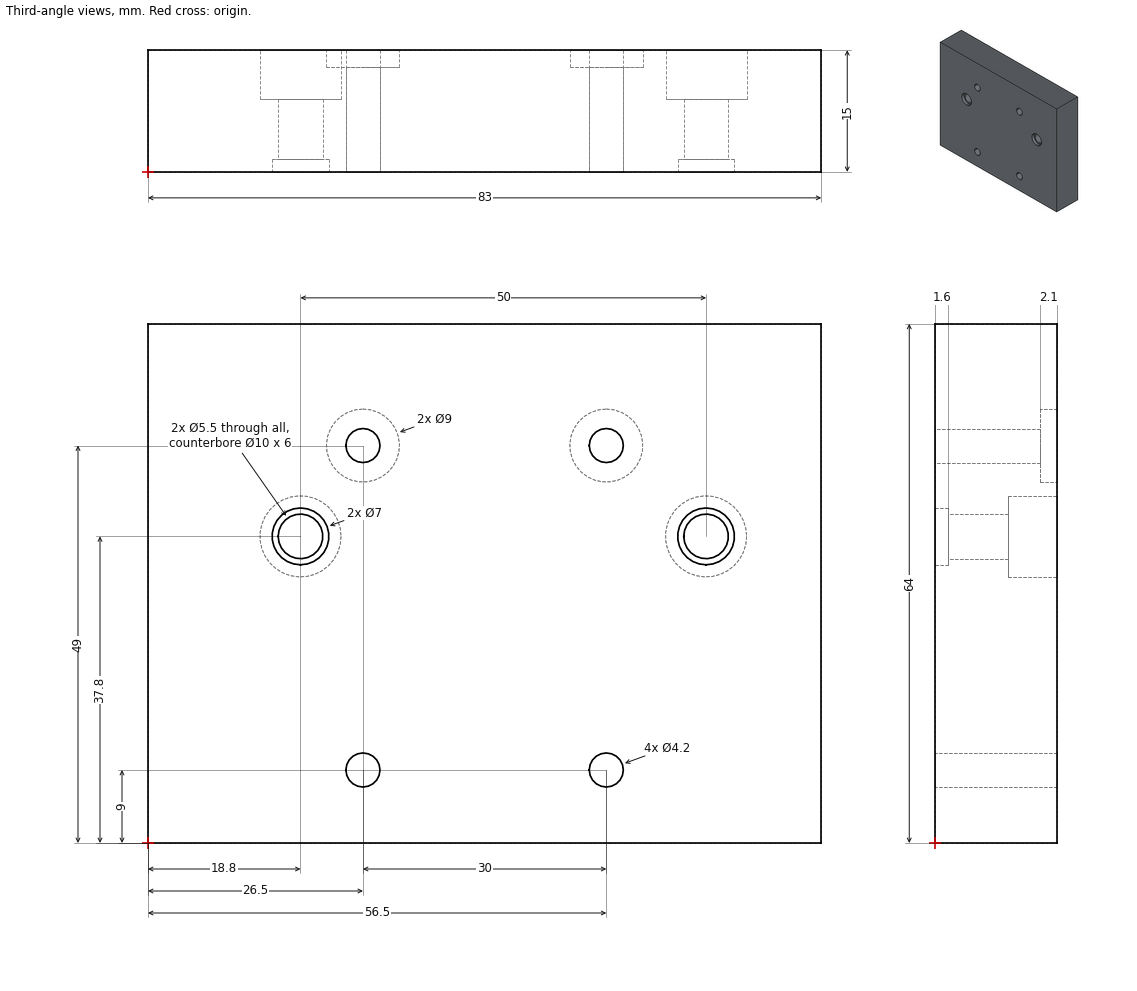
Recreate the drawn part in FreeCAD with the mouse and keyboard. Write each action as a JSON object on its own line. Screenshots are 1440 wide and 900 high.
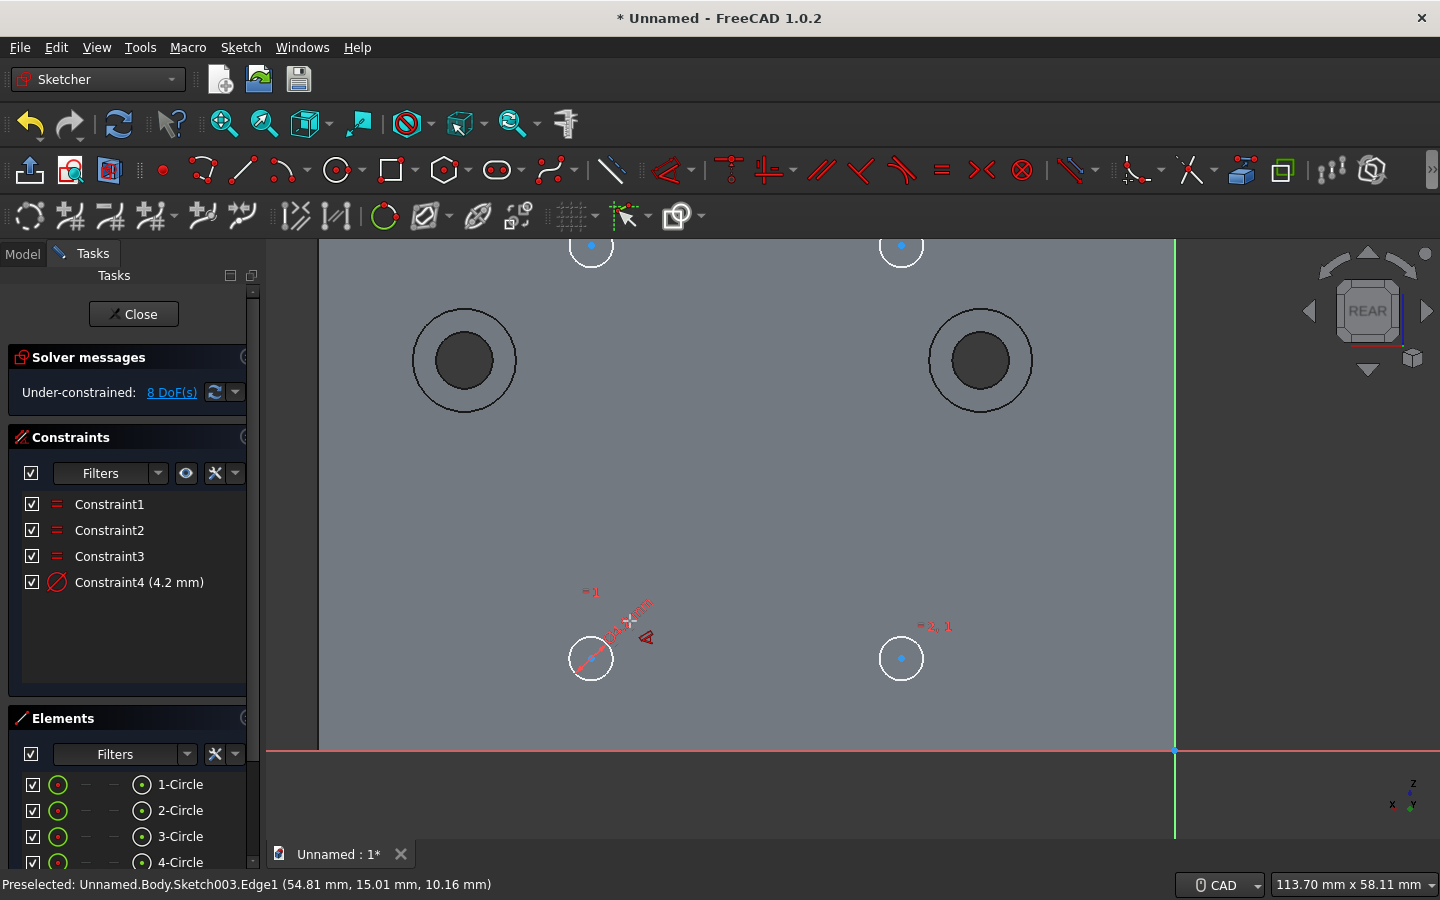
{"action": "left_click", "coordinate": [591, 659]}
{"action": "left_click", "coordinate": [1209, 705]}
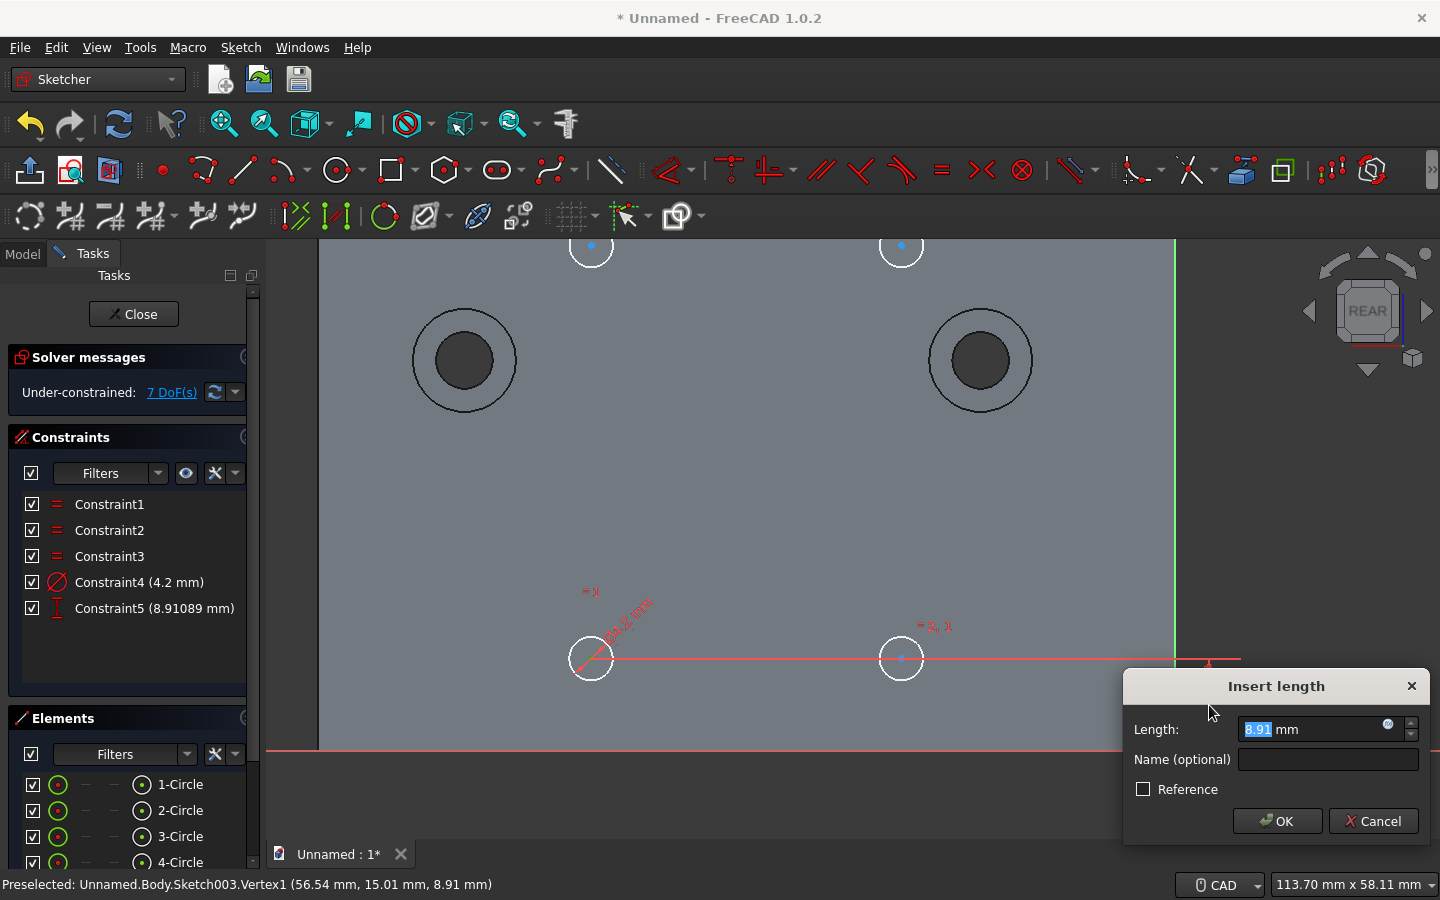
{"action": "type", "text": "9"}
{"action": "key", "text": "Return"}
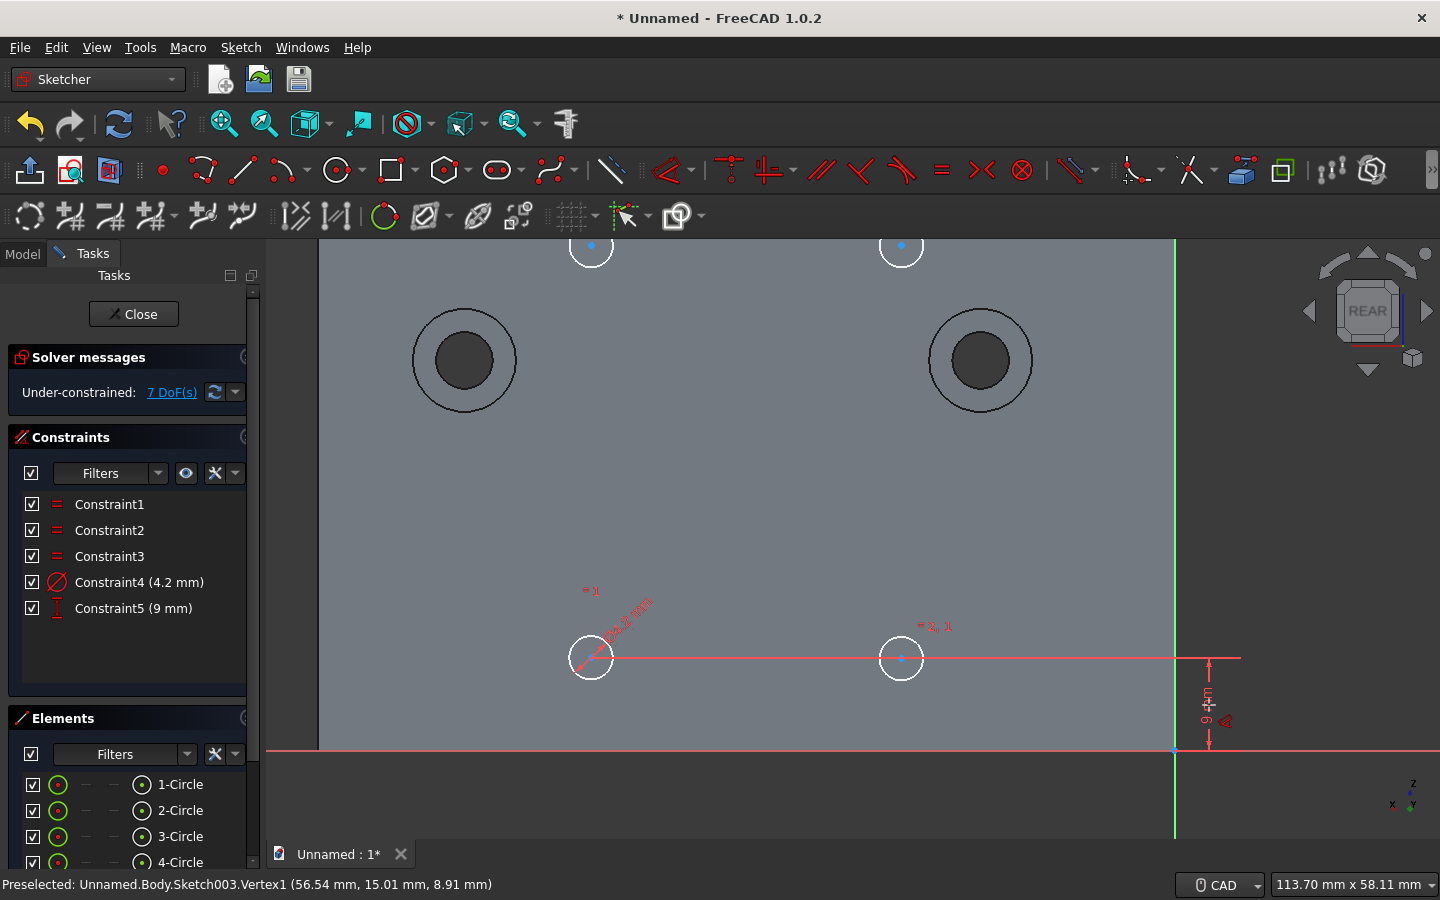
{"action": "left_click", "coordinate": [901, 659]}
{"action": "left_click", "coordinate": [1209, 684]}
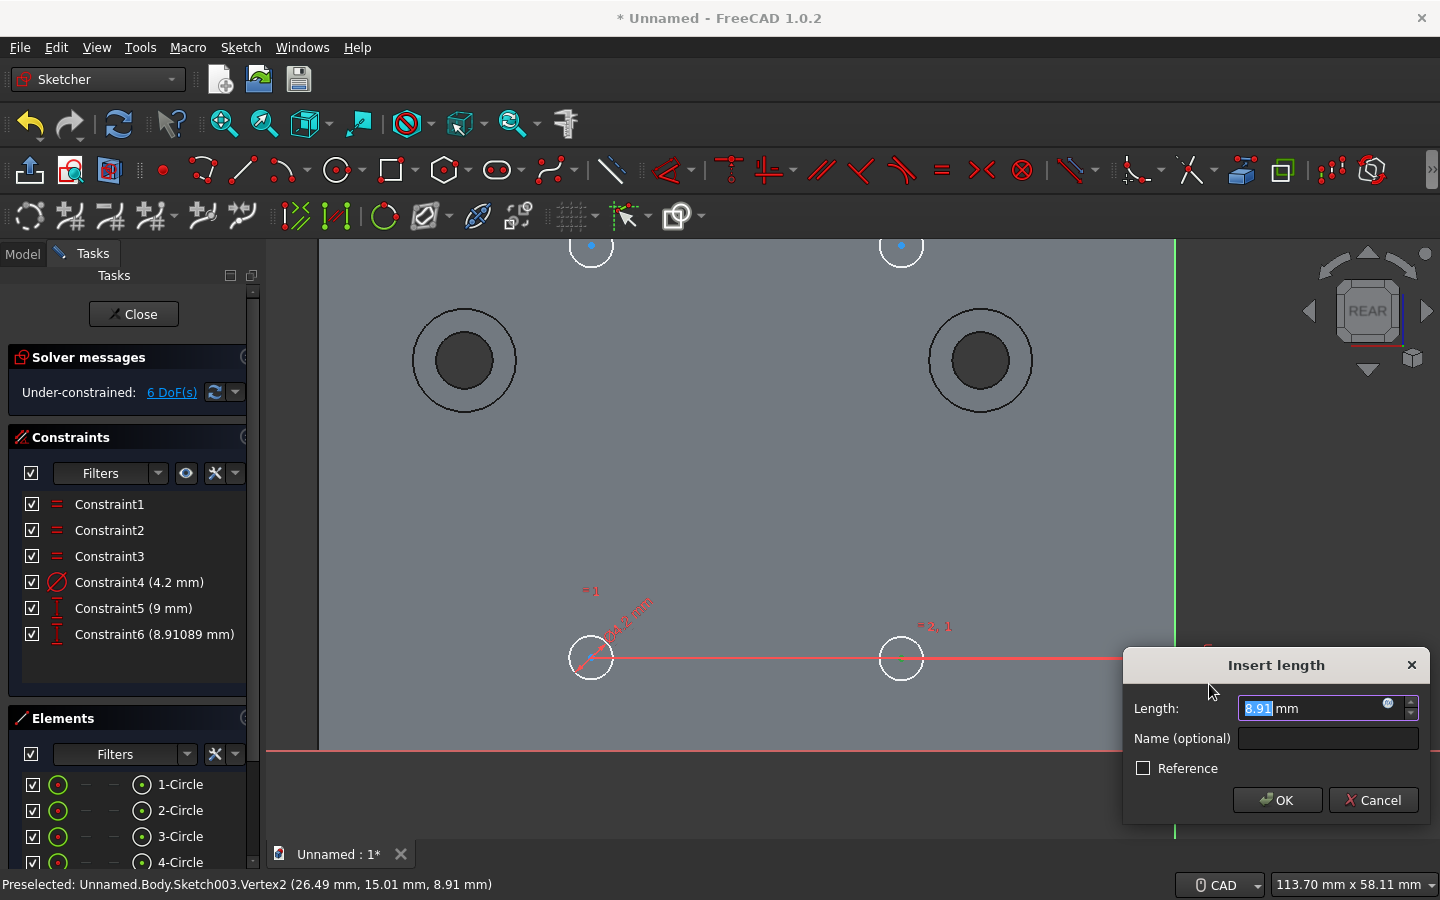
{"action": "type", "text": "9"}
{"action": "key", "text": "Return"}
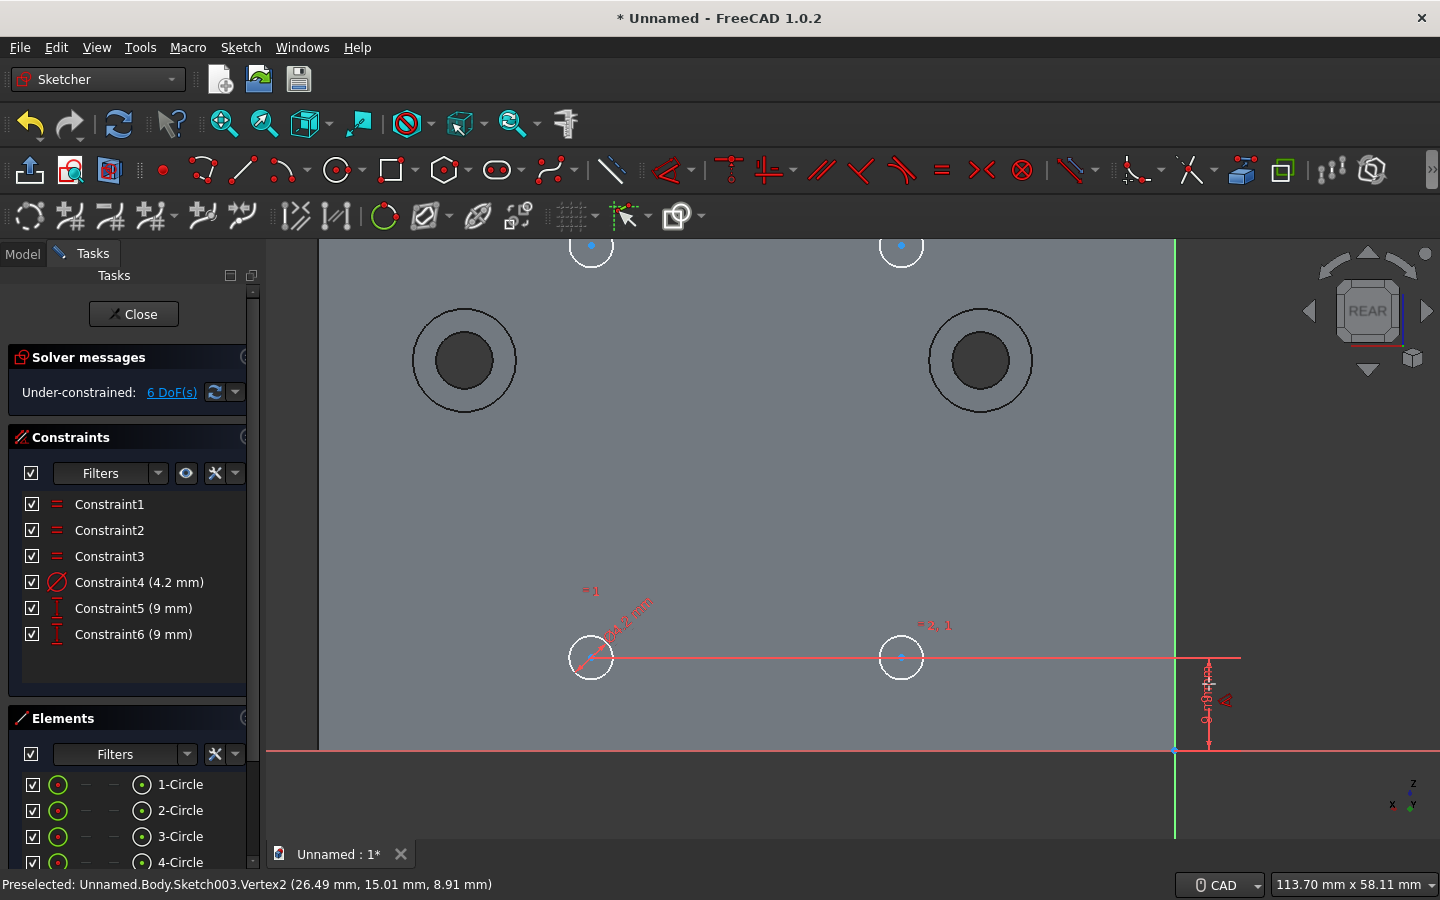
{"action": "scroll", "coordinate": [606, 645], "scroll_direction": "down", "scroll_amount": 2}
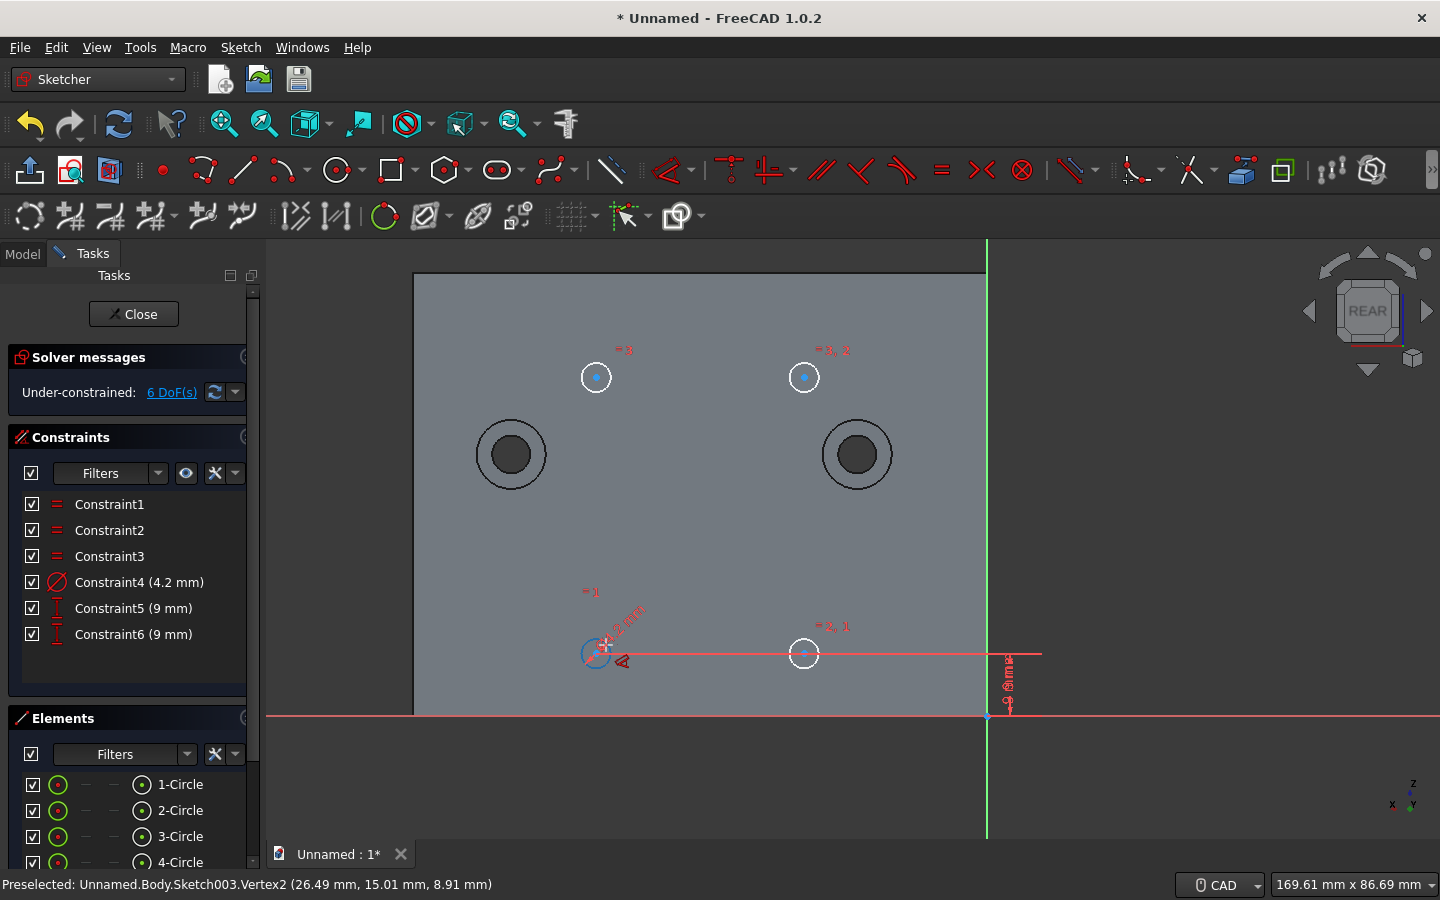
{"action": "left_click", "coordinate": [804, 378]}
{"action": "left_click", "coordinate": [1021, 547]}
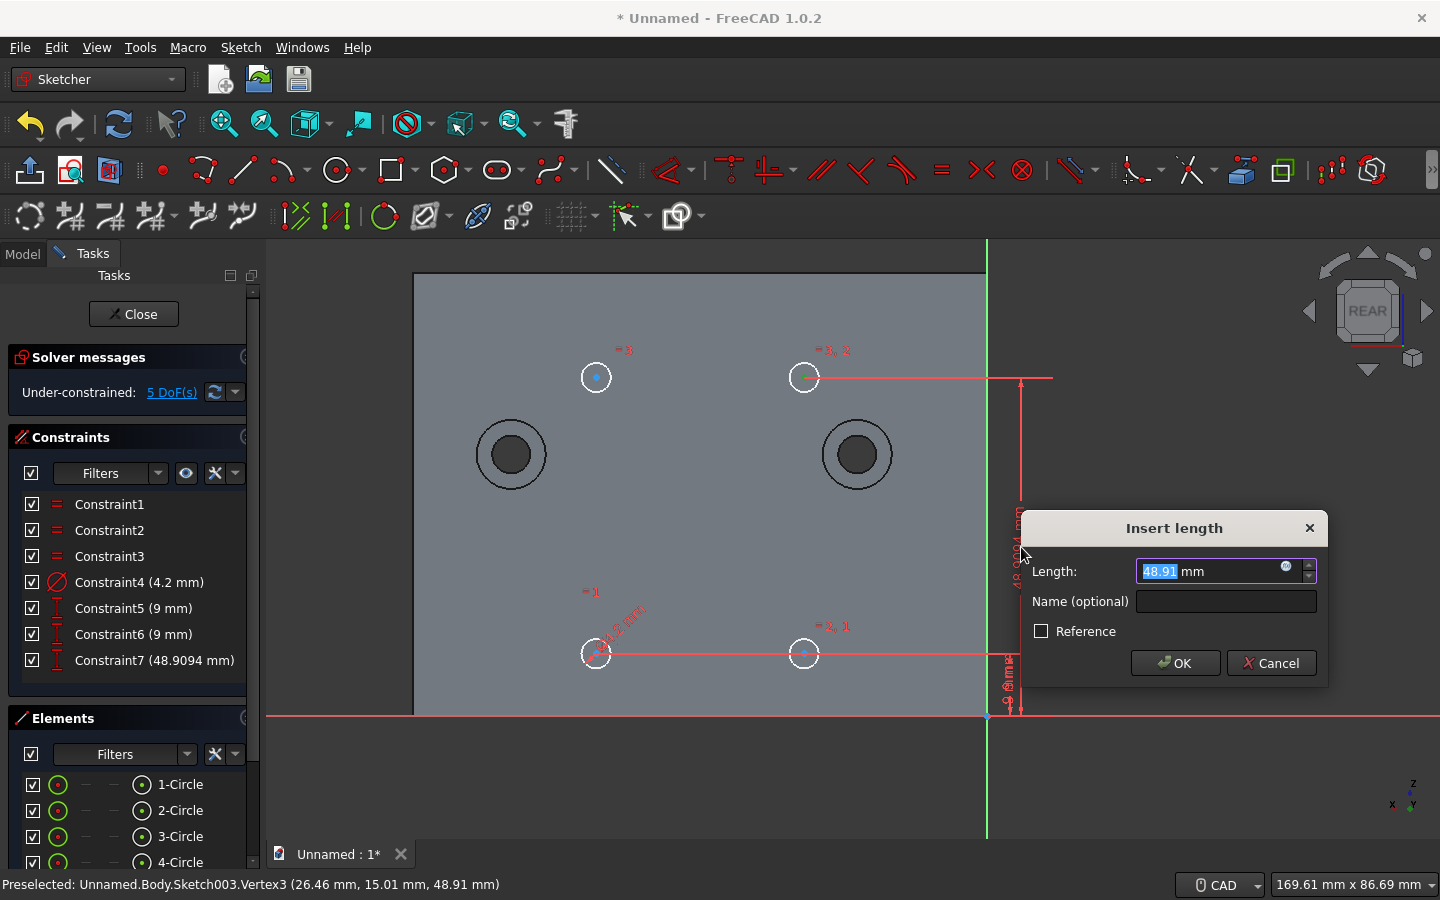
{"action": "type", "text": "49"}
{"action": "key", "text": "Return"}